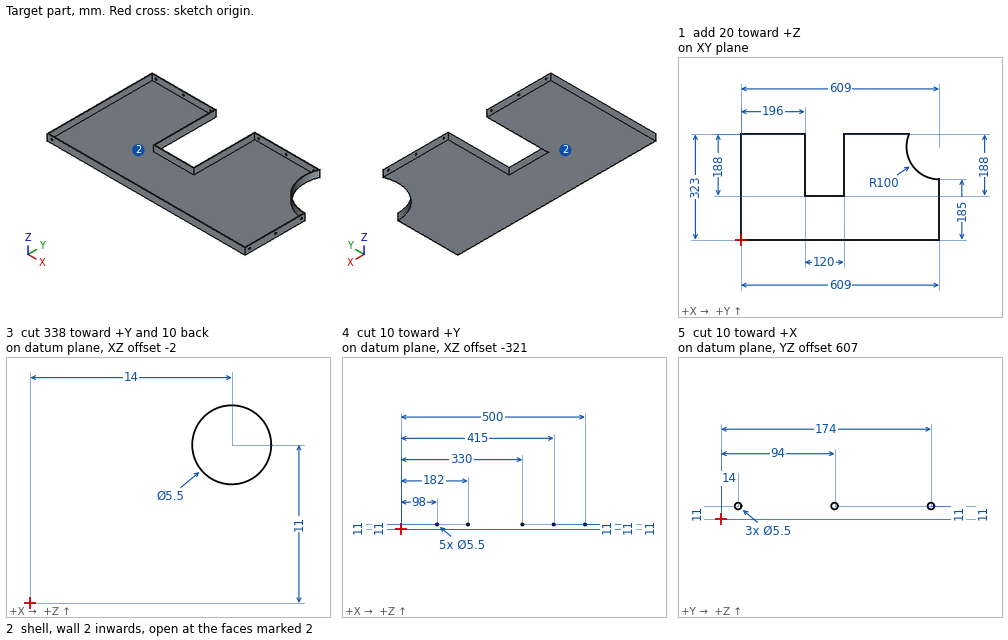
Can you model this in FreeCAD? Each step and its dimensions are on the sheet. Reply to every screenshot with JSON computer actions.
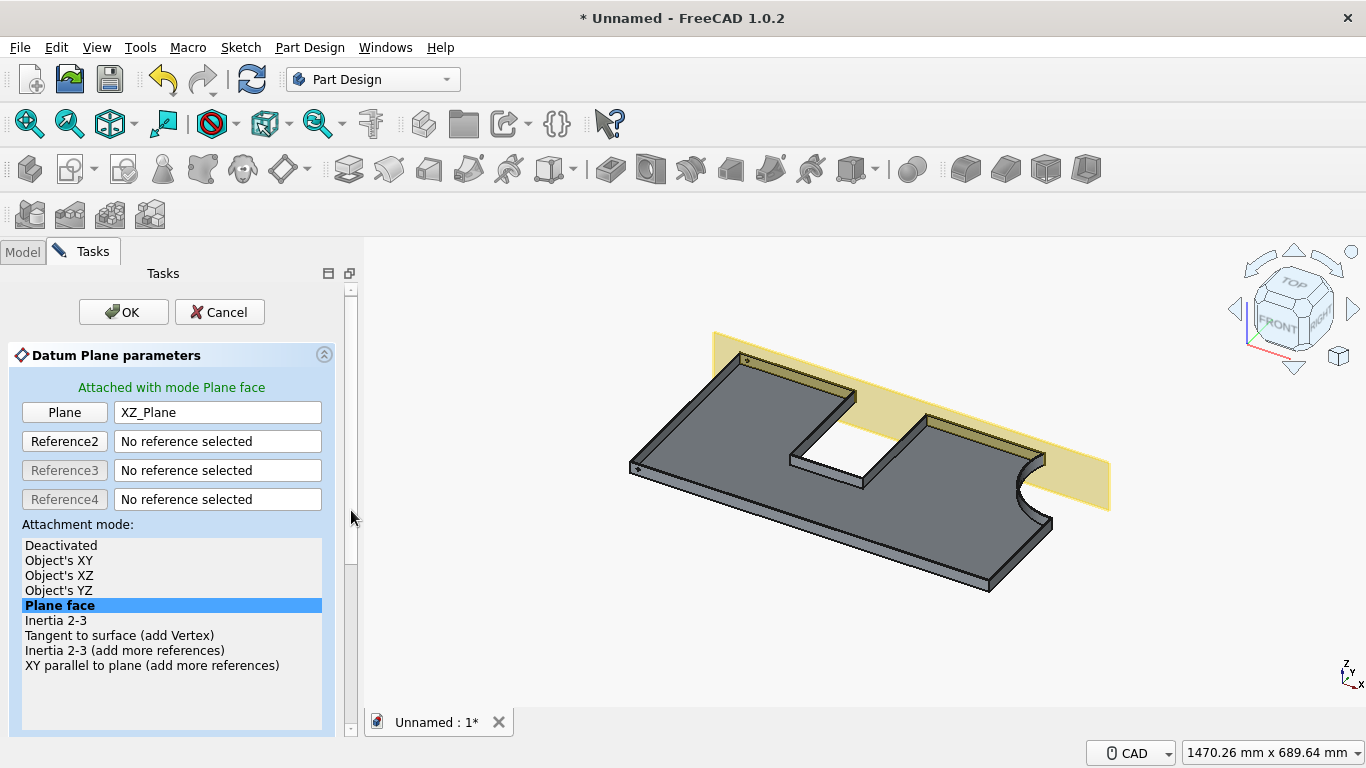
{"action": "left_click", "coordinate": [124, 312]}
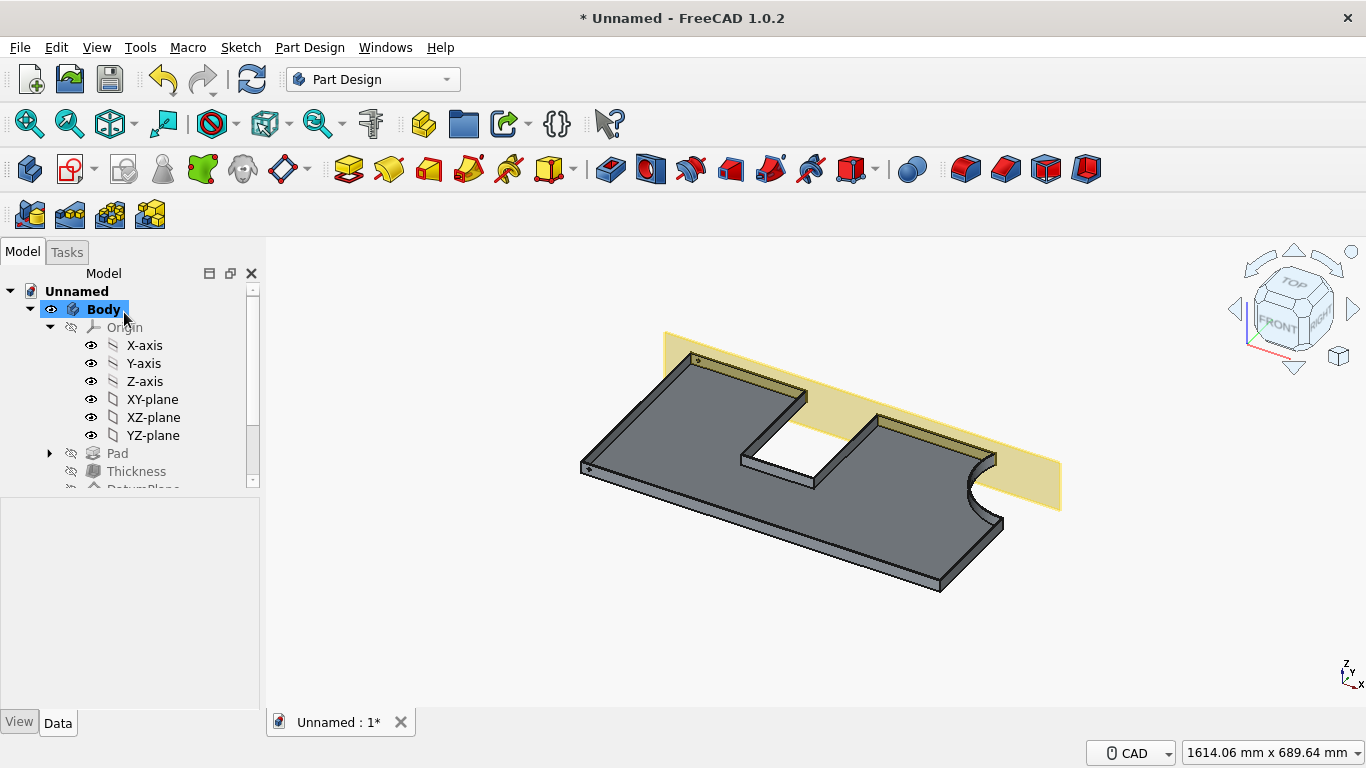
{"action": "scroll", "coordinate": [100, 377], "scroll_direction": "down", "scroll_amount": 3}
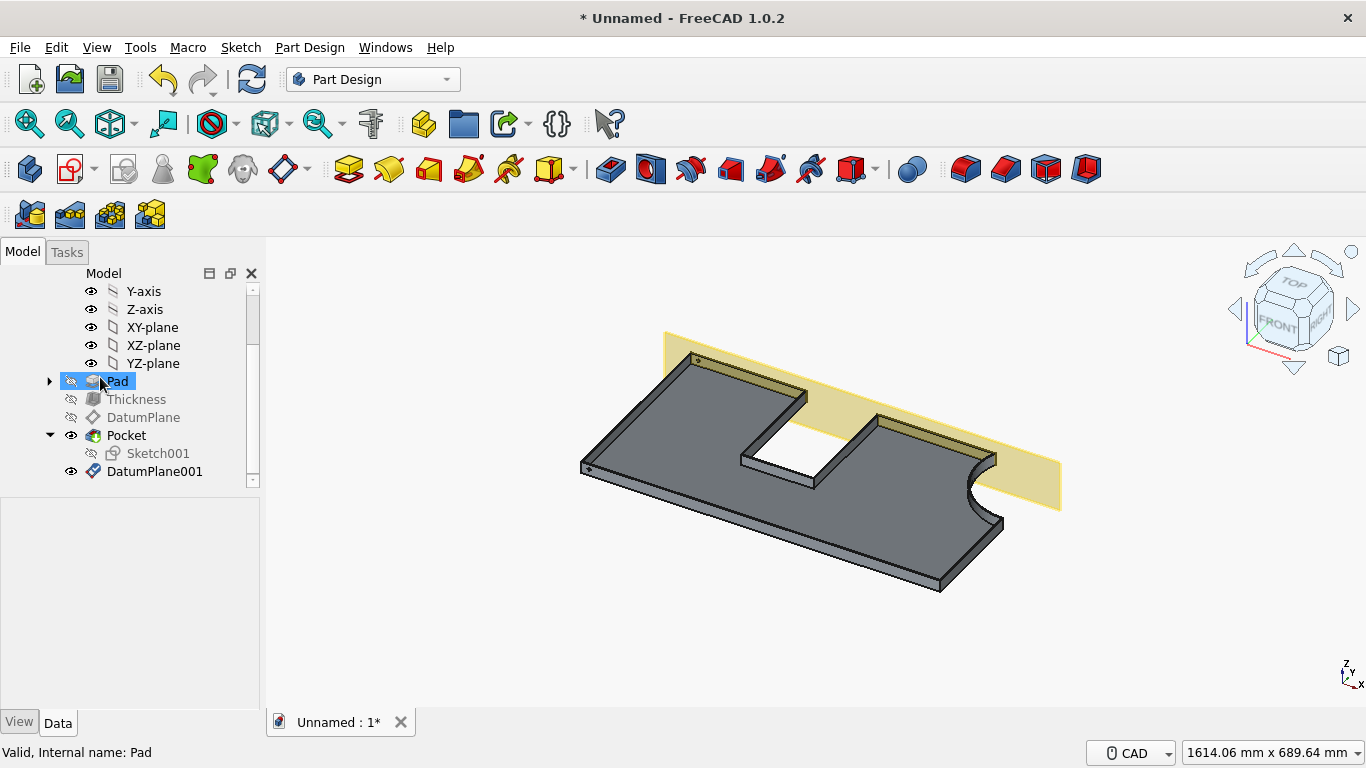
{"action": "left_click", "coordinate": [116, 471]}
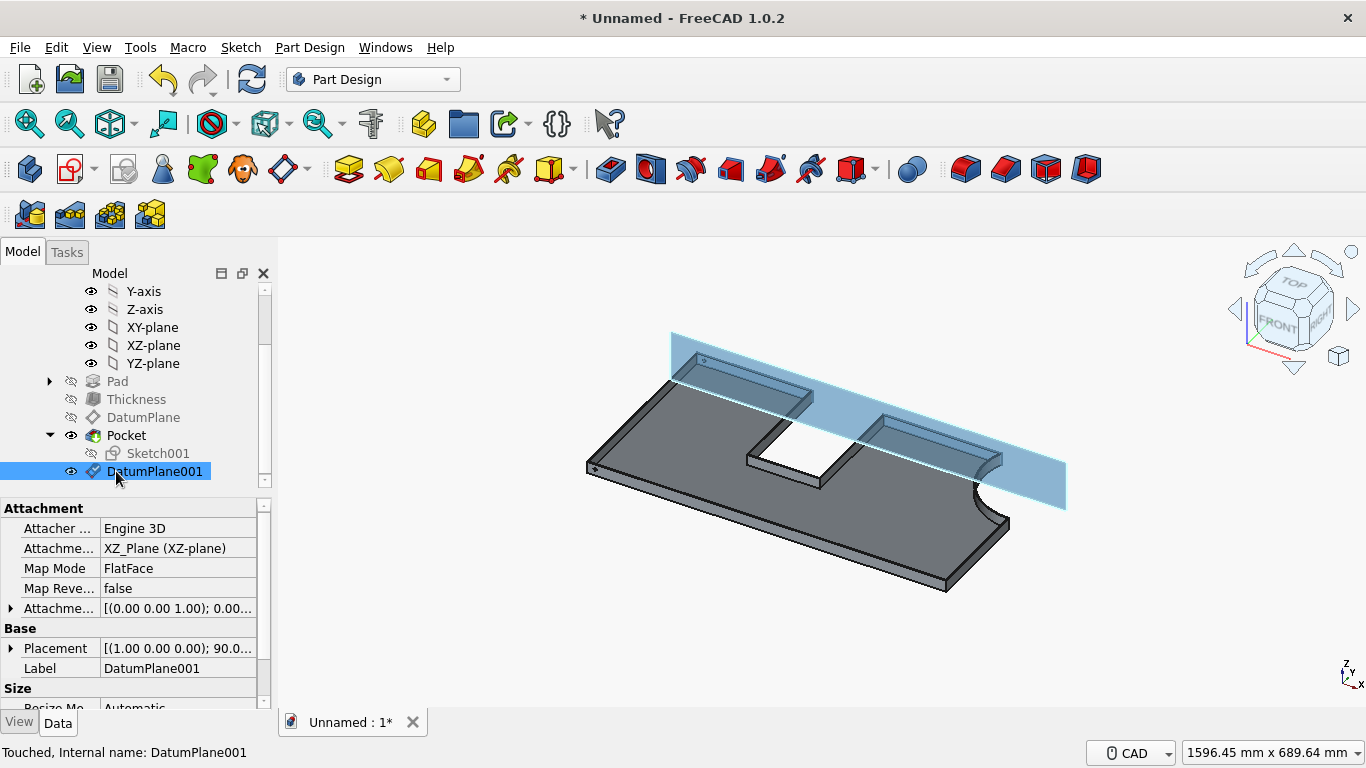
{"action": "left_click", "coordinate": [70, 170]}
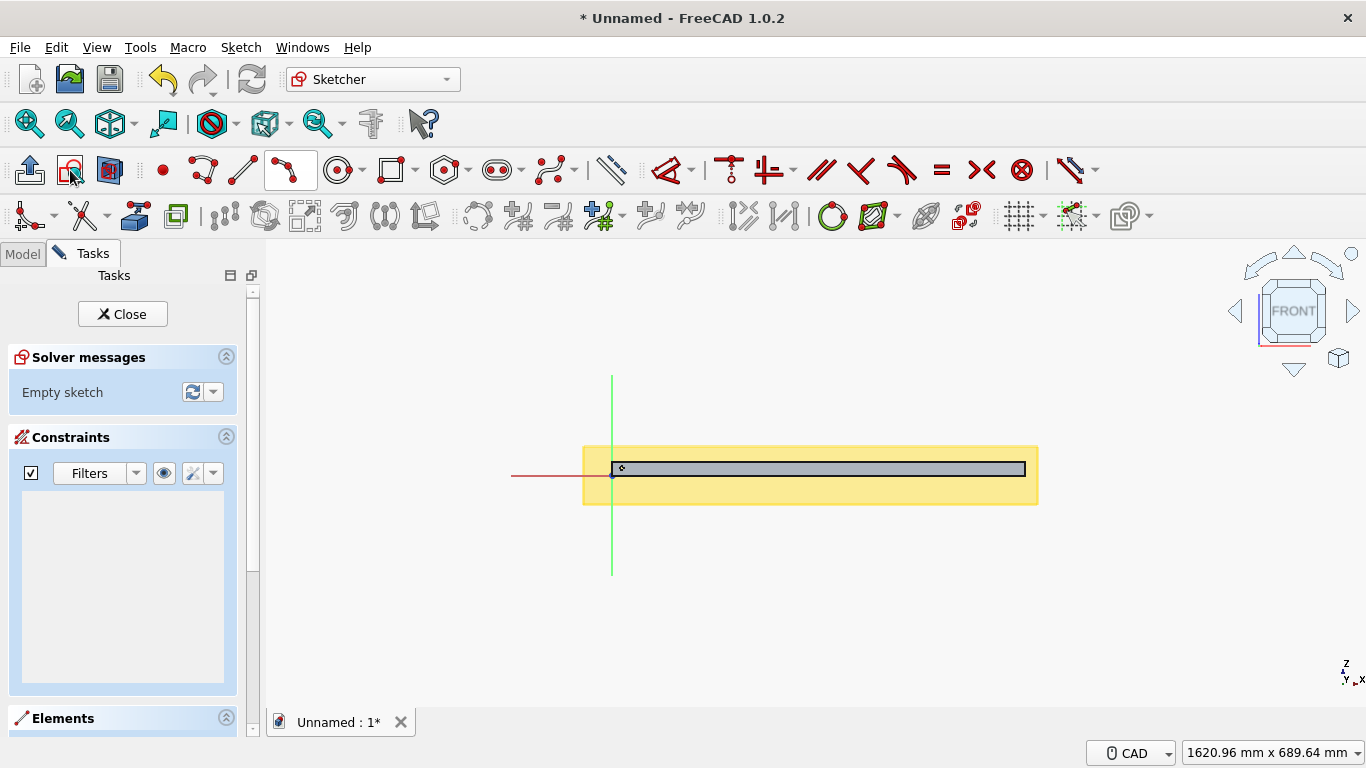
{"action": "left_click", "coordinate": [110, 170]}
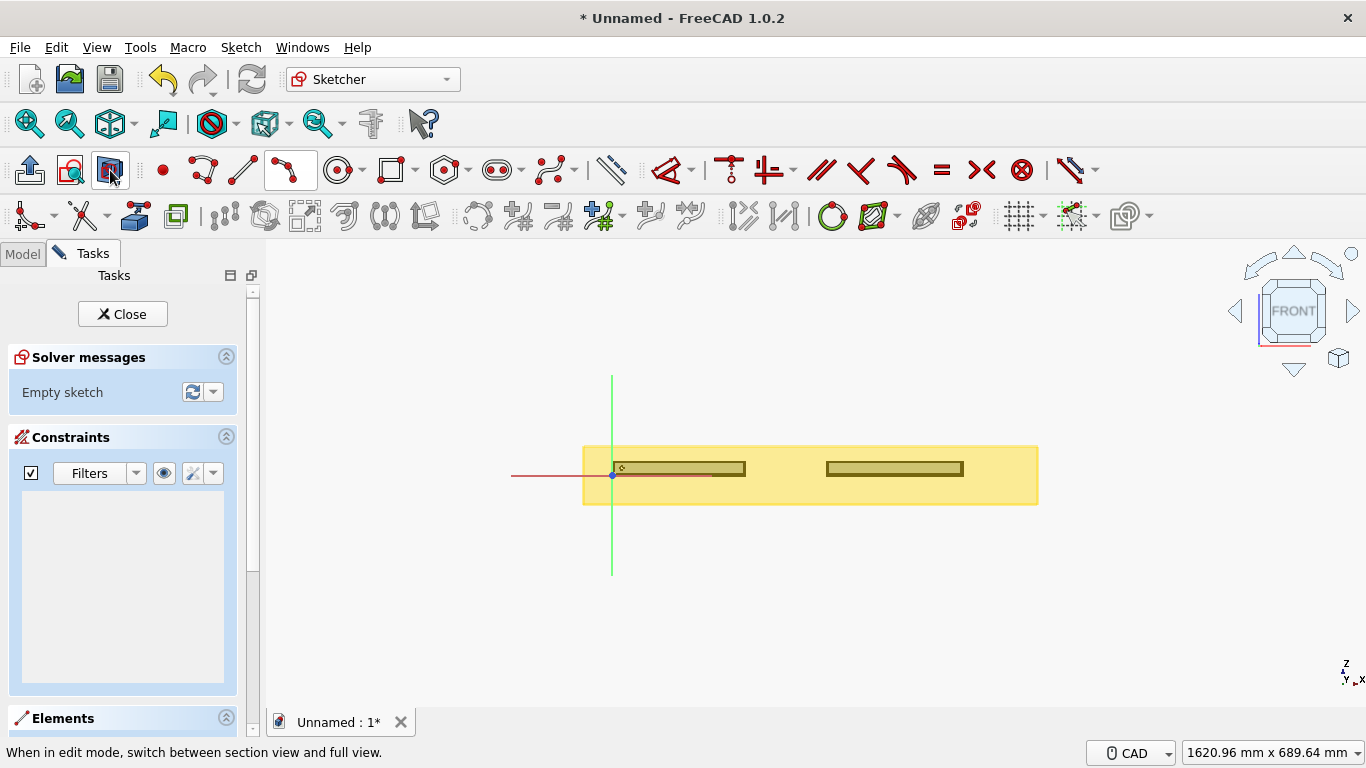
{"action": "scroll", "coordinate": [826, 468], "scroll_direction": "up", "scroll_amount": 3}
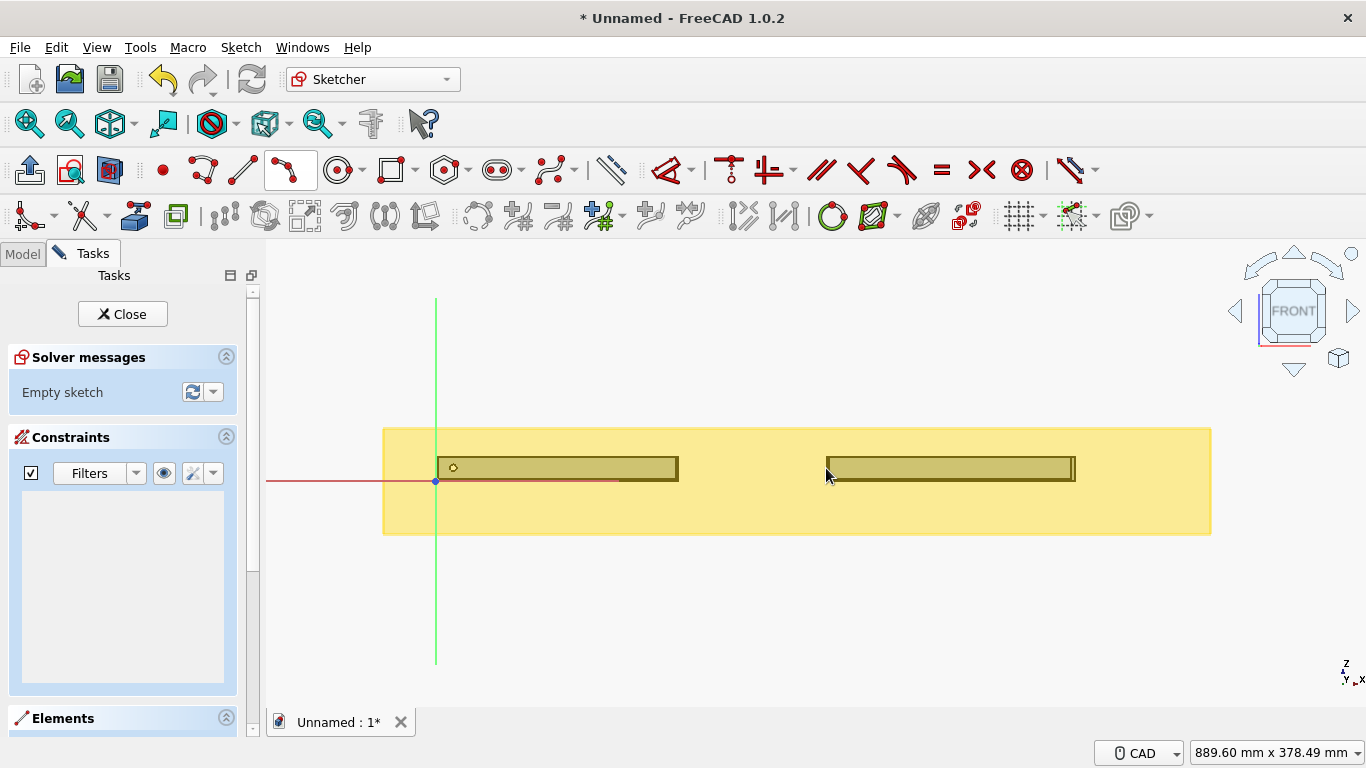
{"action": "key", "text": "g c"}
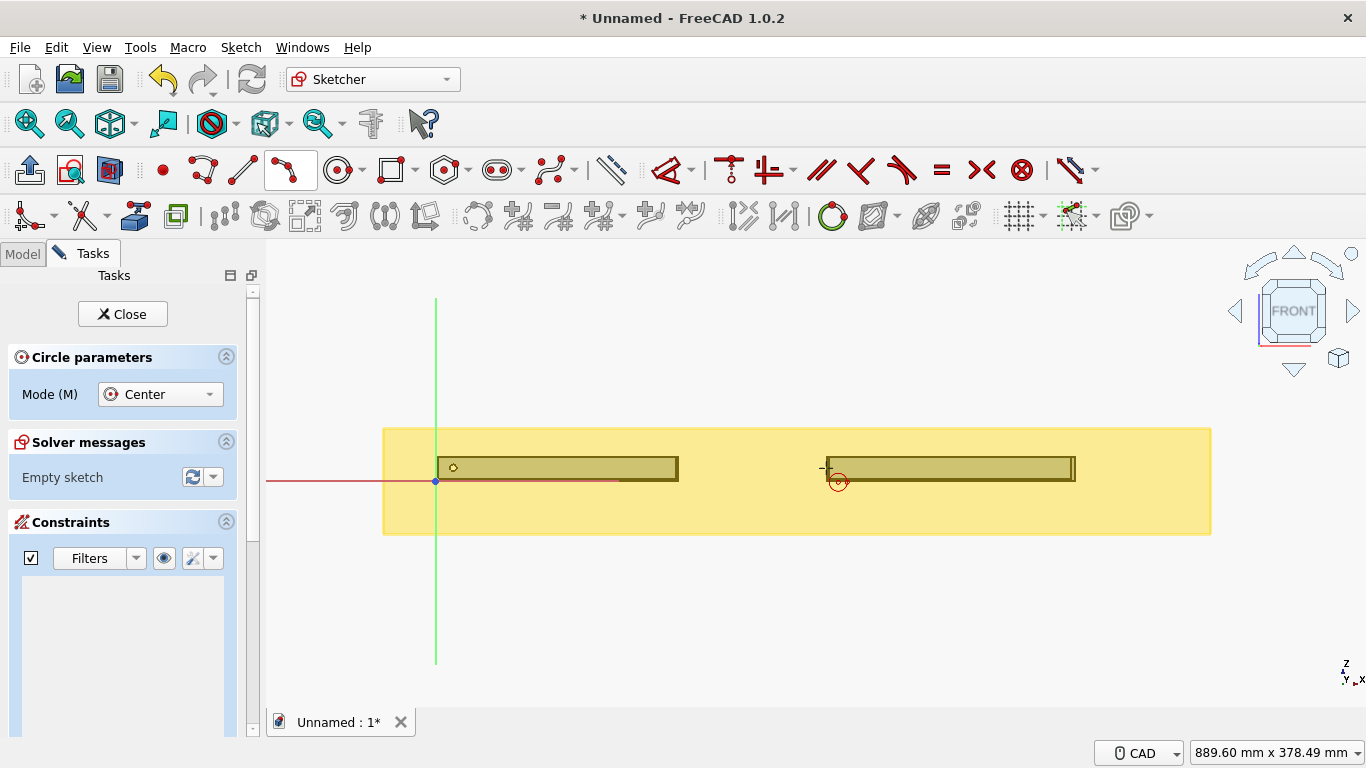
{"action": "scroll", "coordinate": [557, 468], "scroll_direction": "up", "scroll_amount": 10}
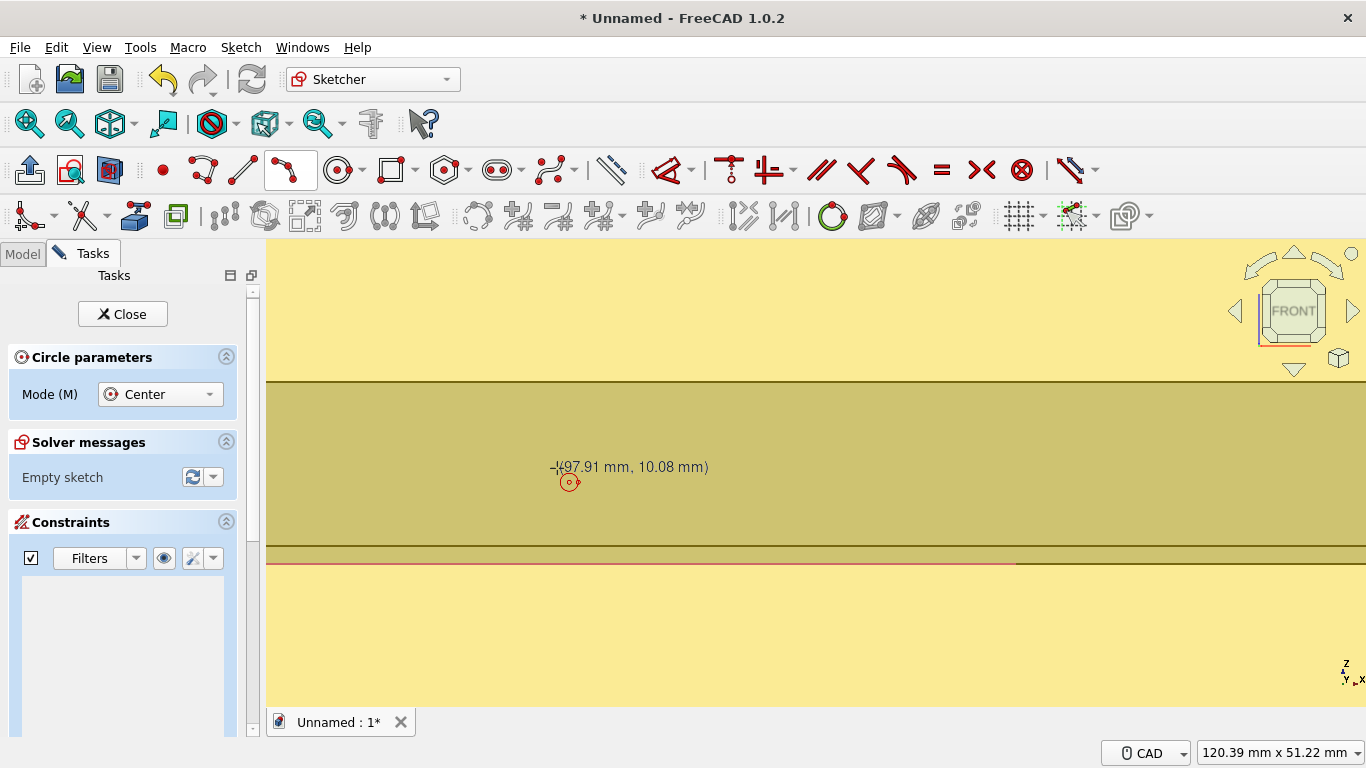
{"action": "scroll", "coordinate": [558, 469], "scroll_direction": "down", "scroll_amount": 10}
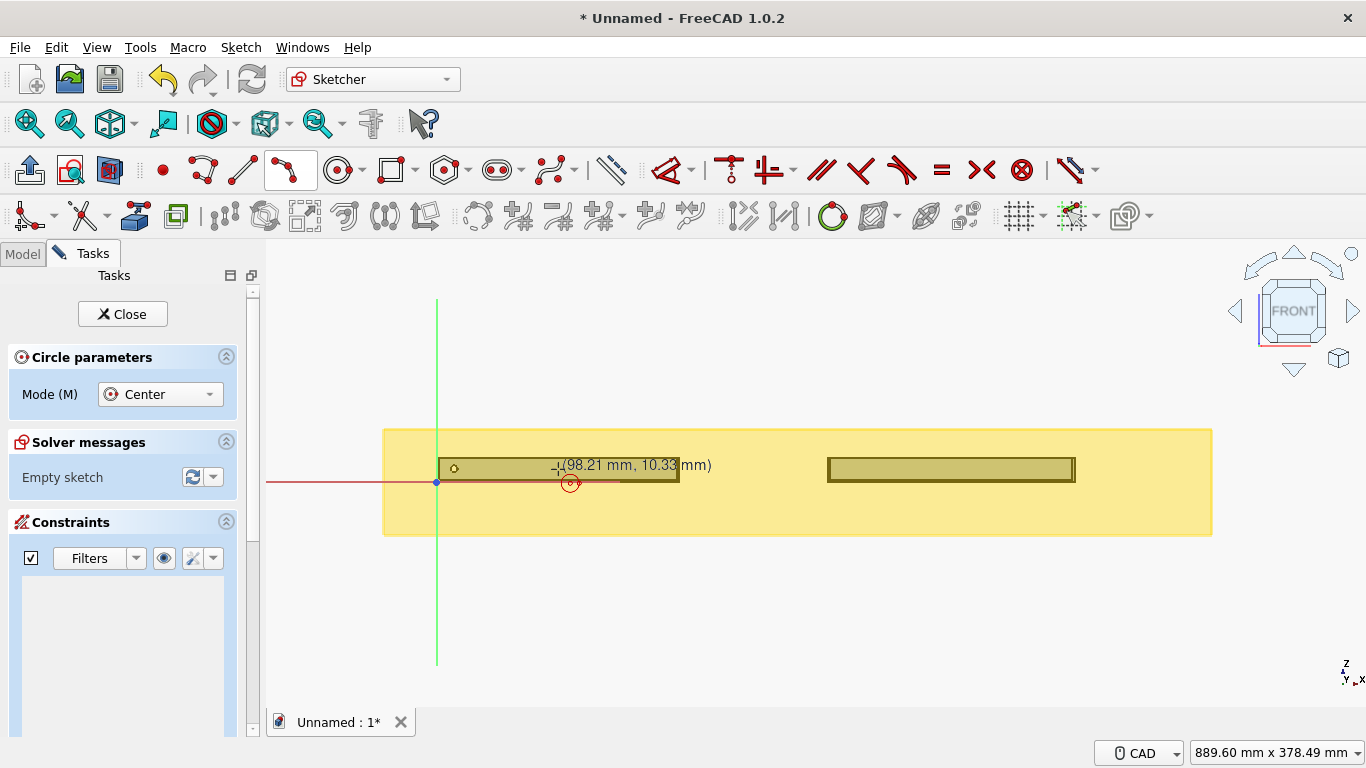
{"action": "left_click", "coordinate": [558, 469]}